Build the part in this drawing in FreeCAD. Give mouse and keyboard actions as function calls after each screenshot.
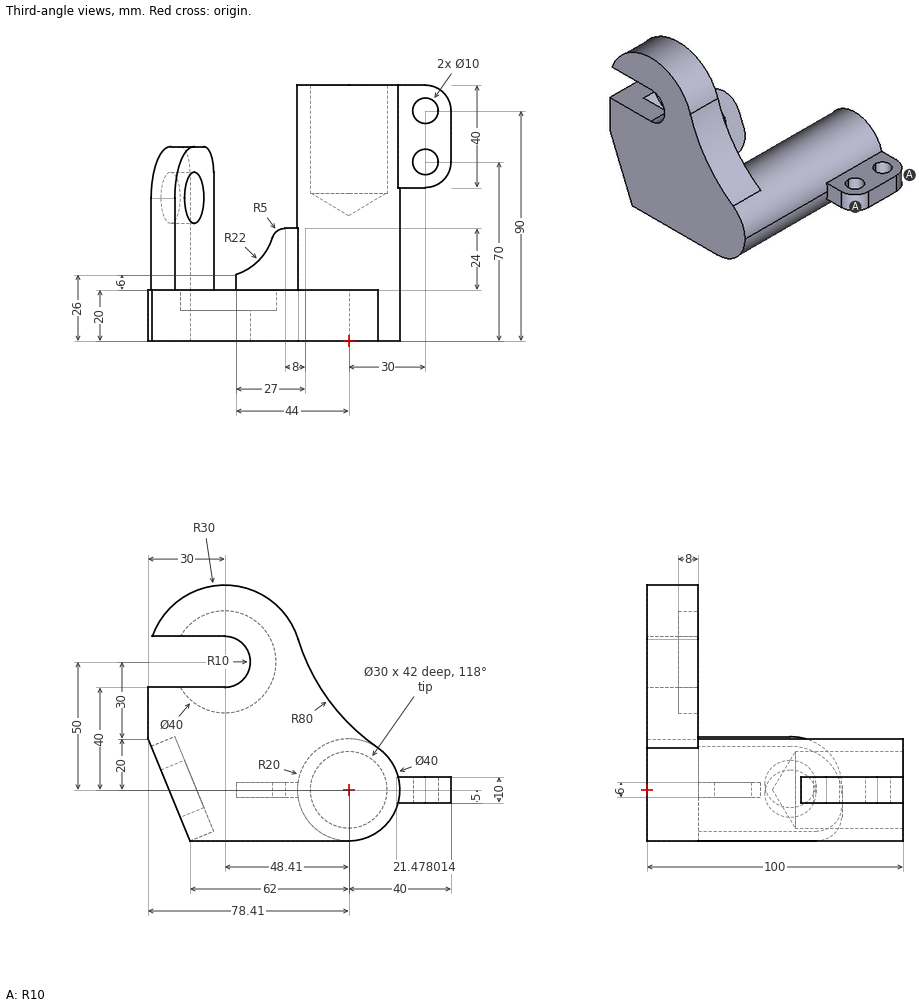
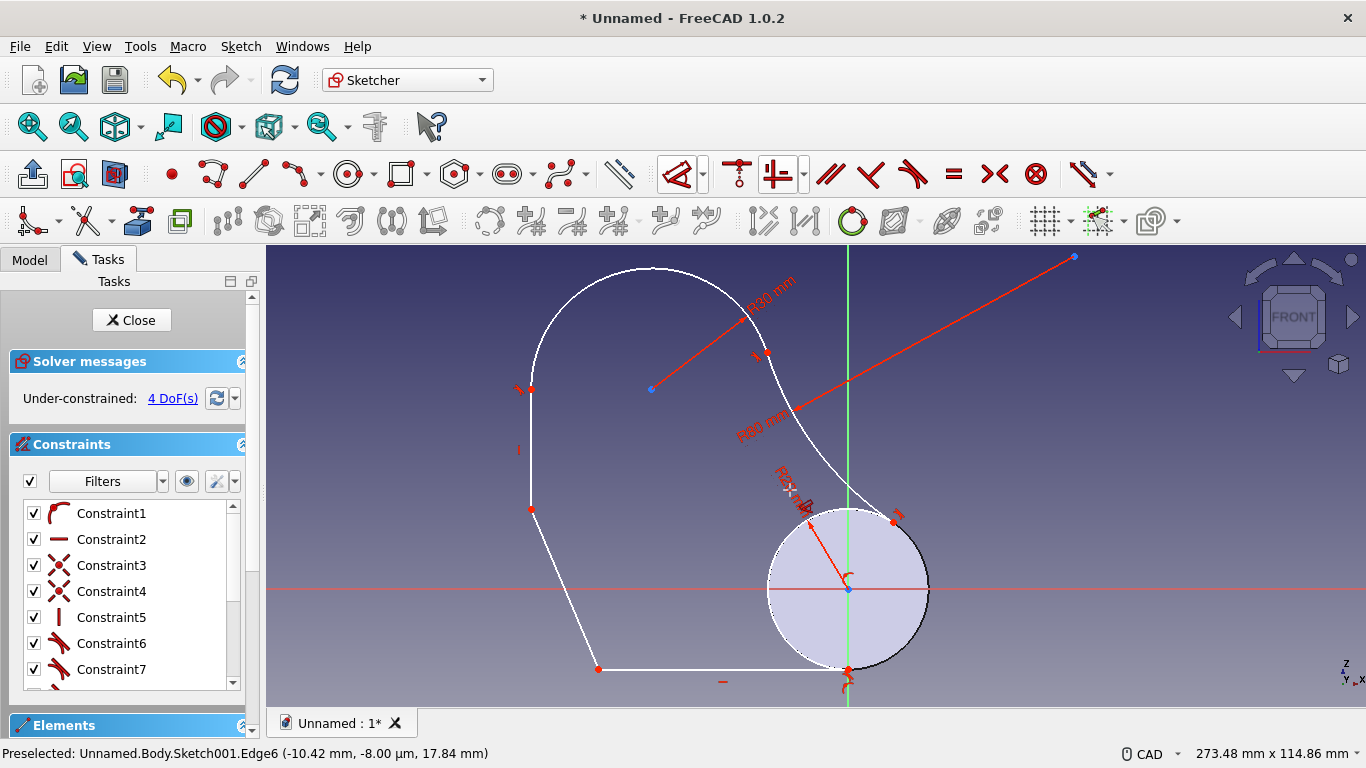
click(774, 670)
click(724, 636)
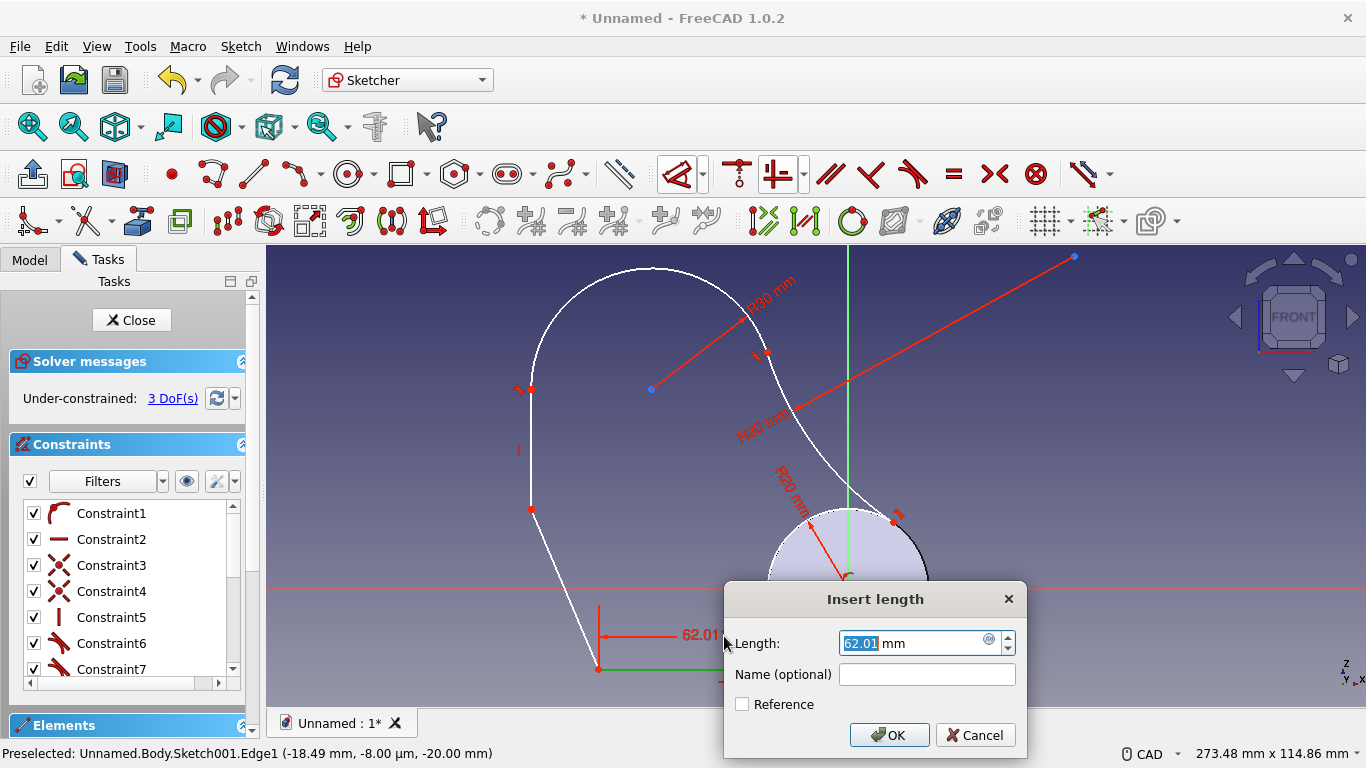
text(62)
key(Return)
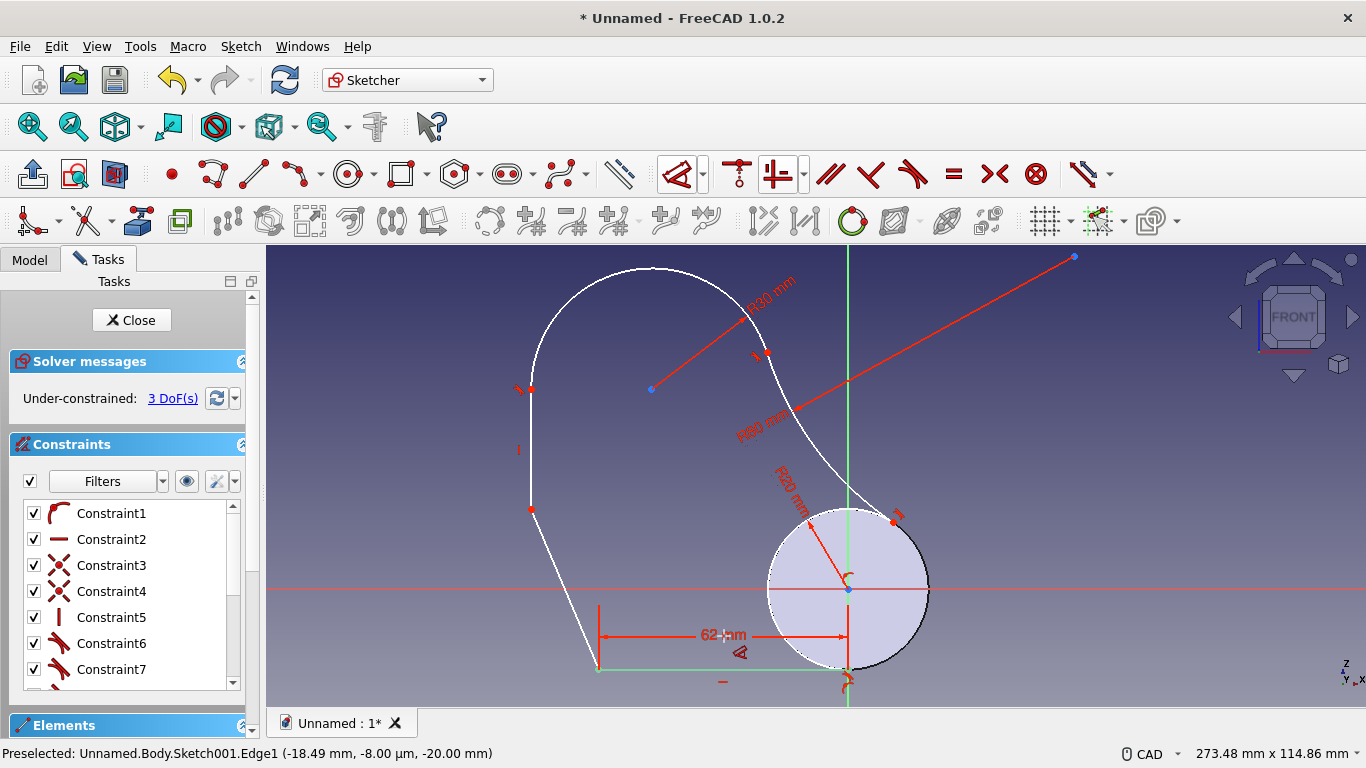
click(531, 474)
click(497, 450)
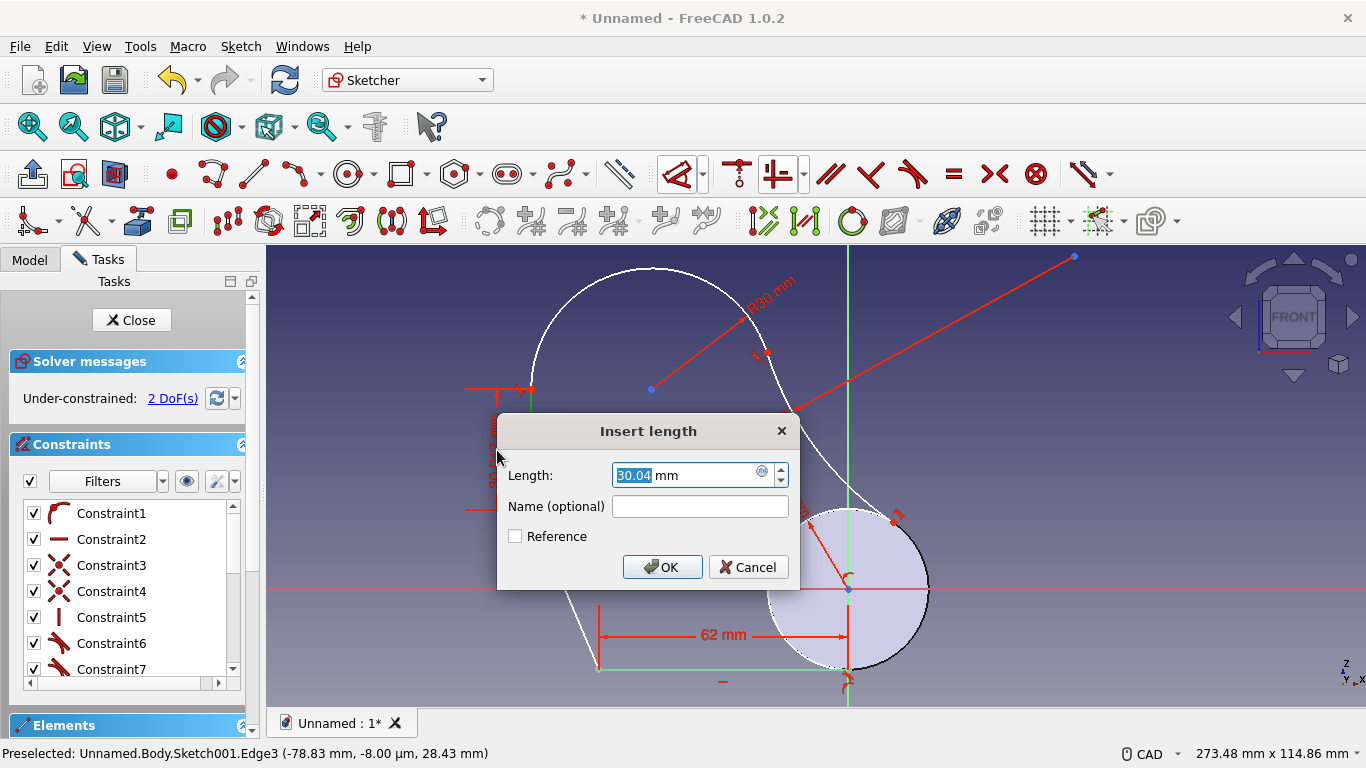
text(30)
key(Return)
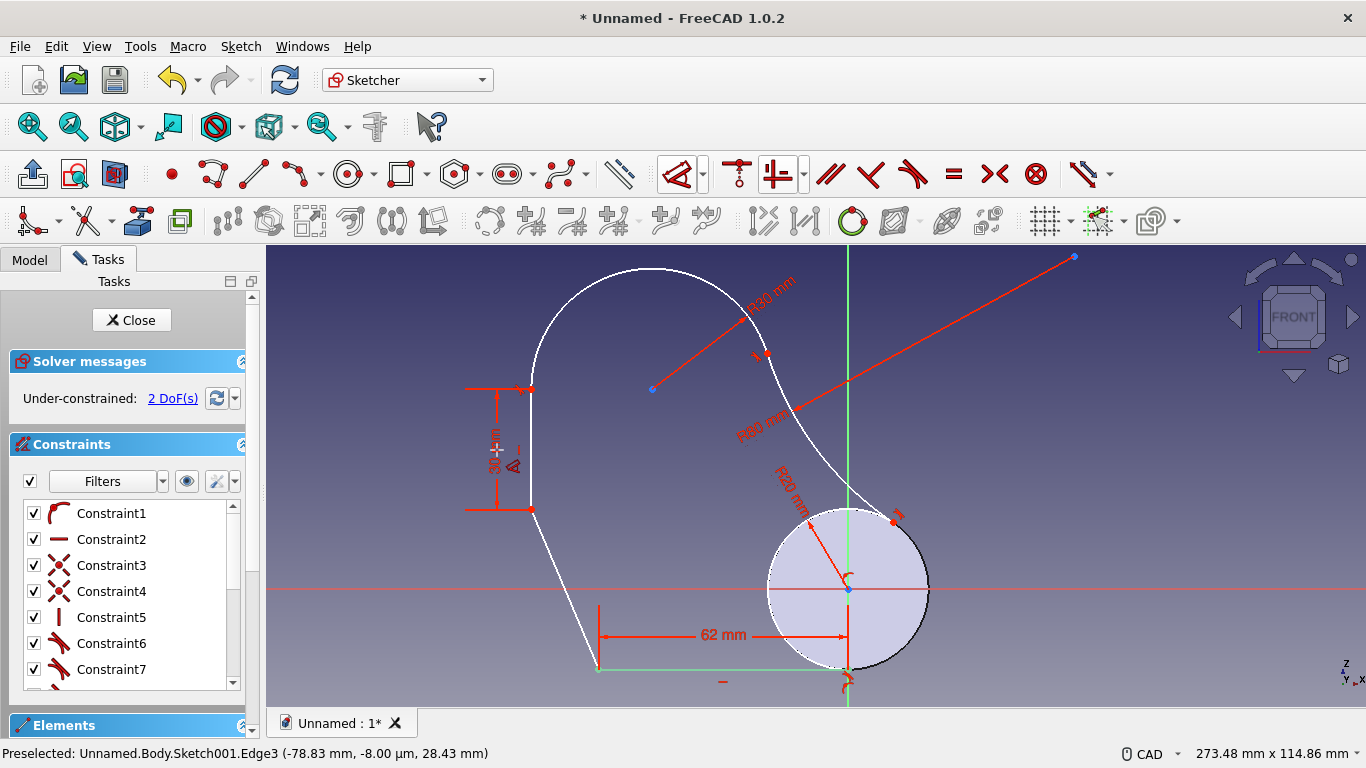
click(531, 510)
click(497, 550)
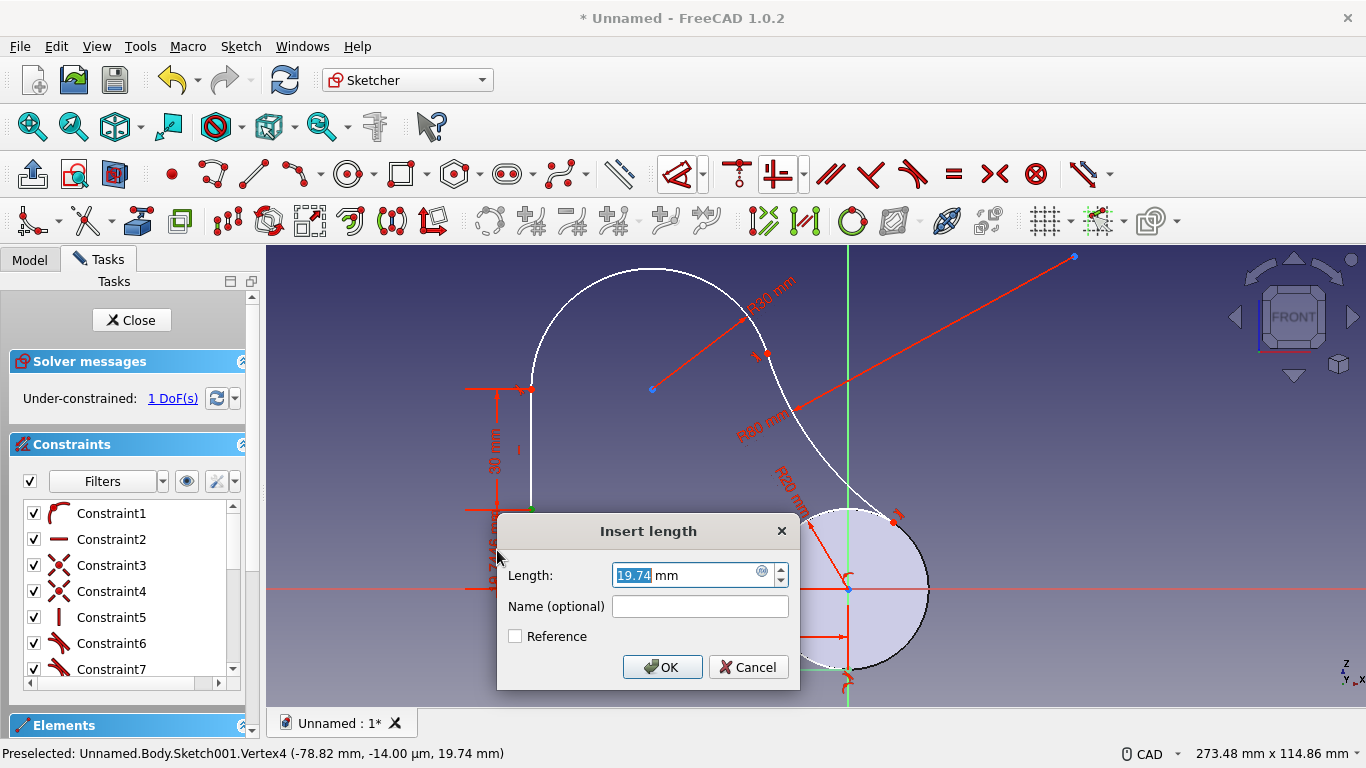
text(20)
key(Return)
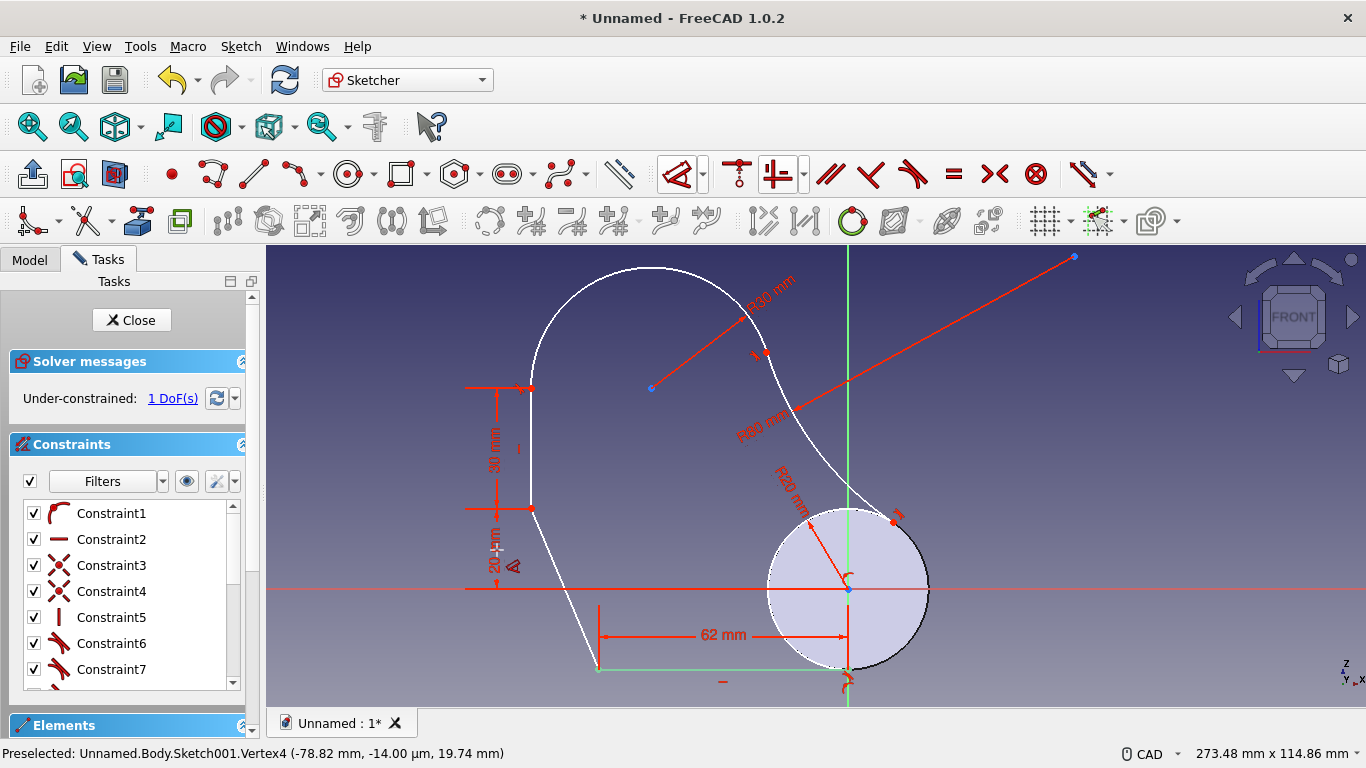
click(531, 509)
click(617, 623)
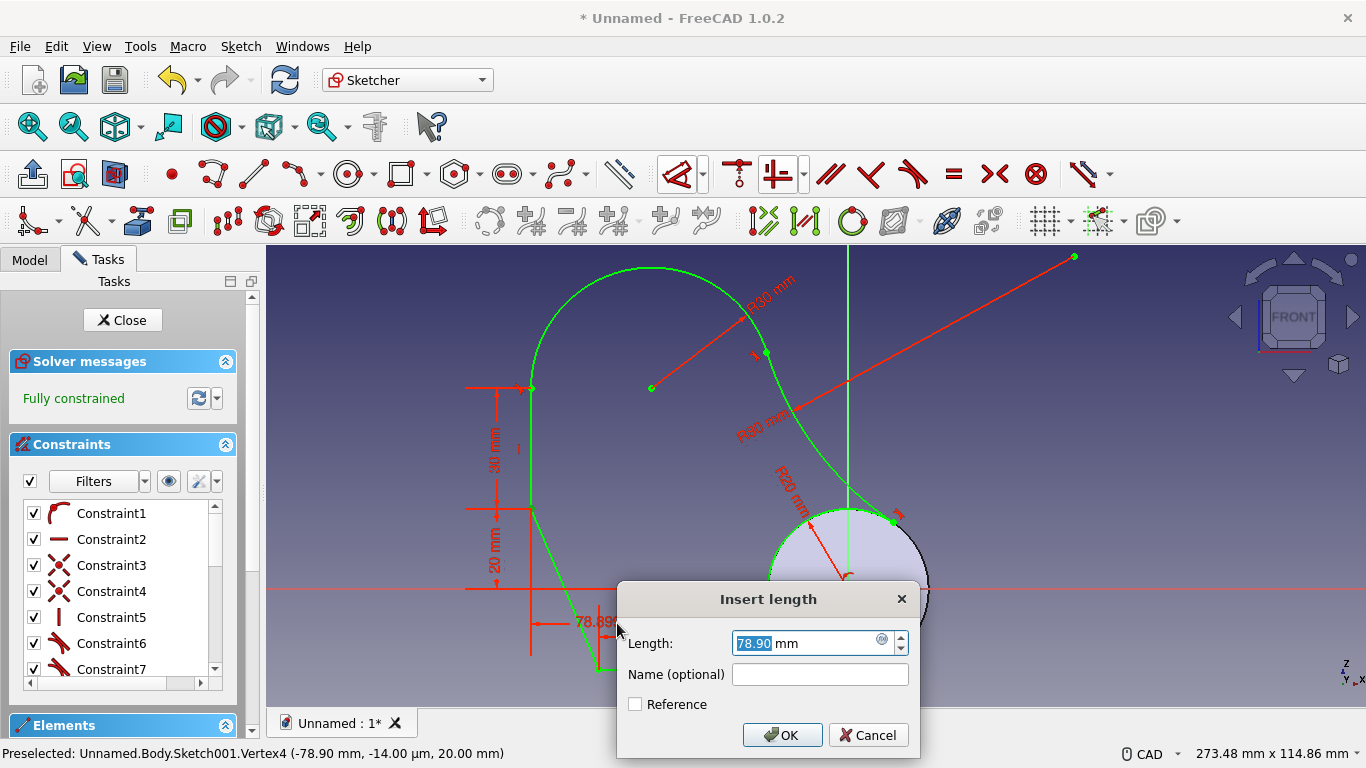
text(78.41)
key(Return)
key(Escape)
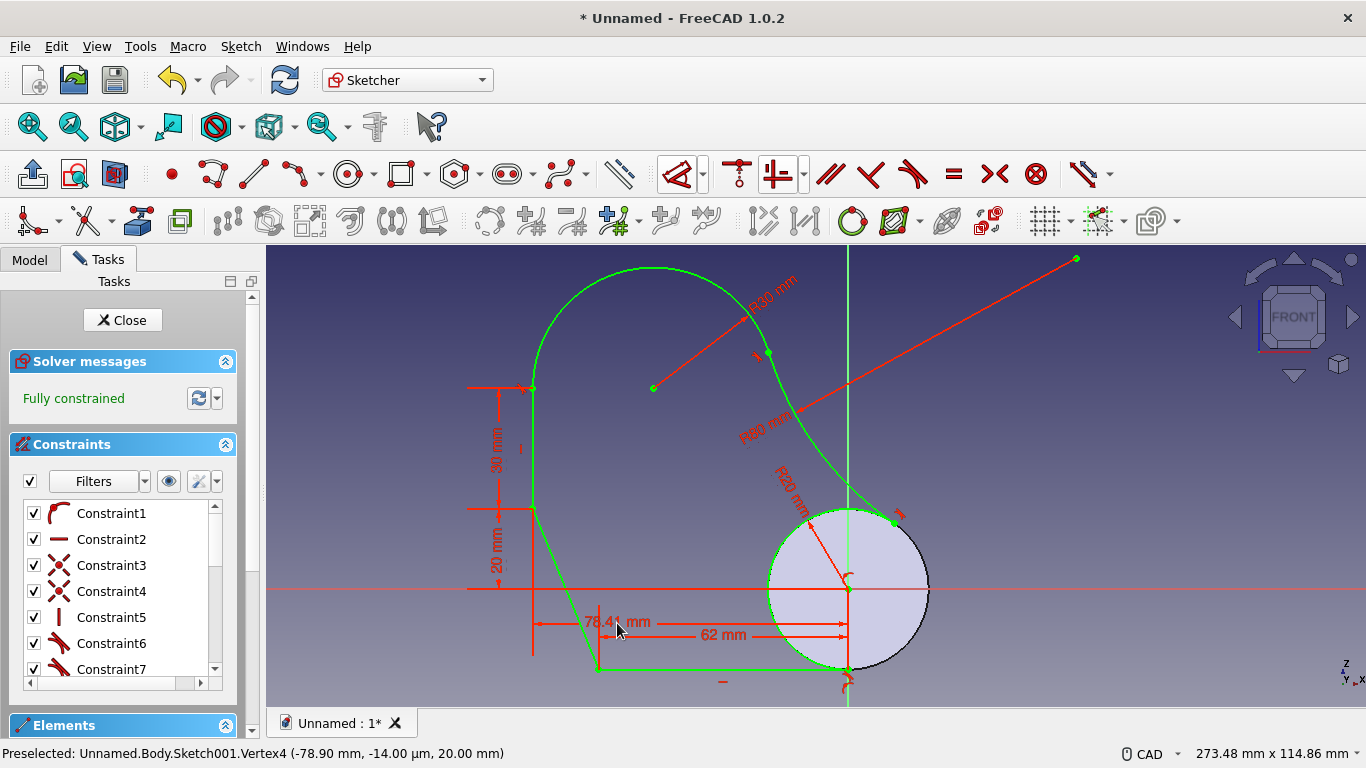
click(123, 320)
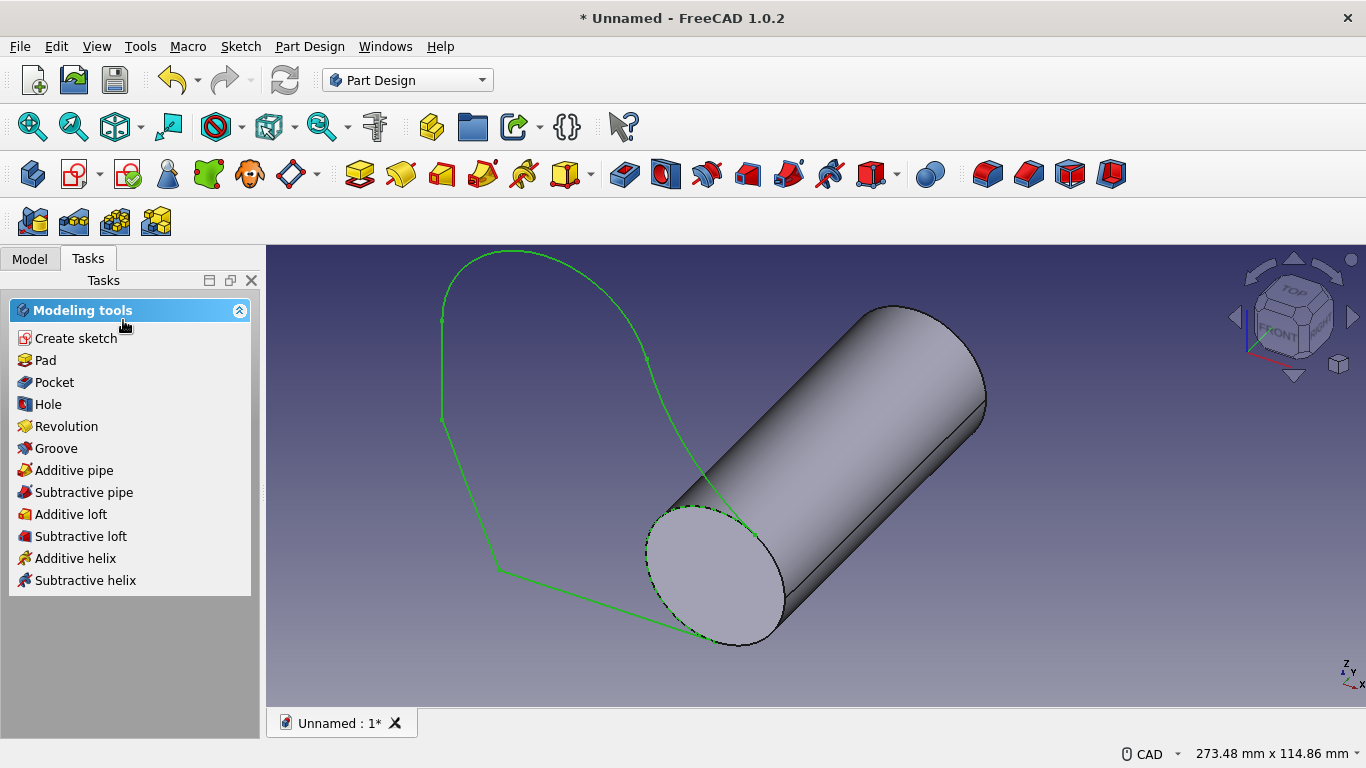
click(360, 174)